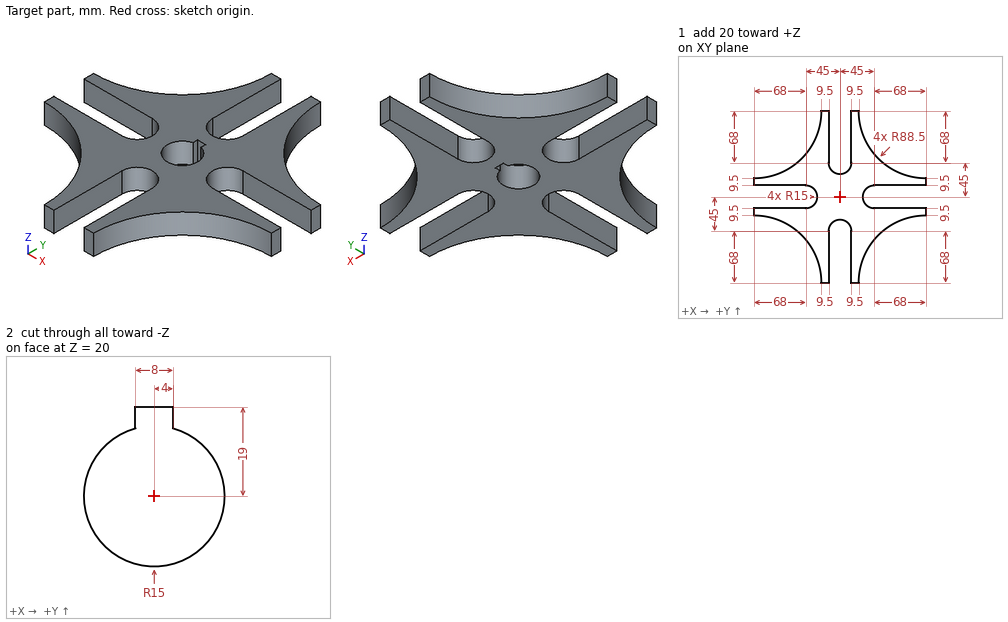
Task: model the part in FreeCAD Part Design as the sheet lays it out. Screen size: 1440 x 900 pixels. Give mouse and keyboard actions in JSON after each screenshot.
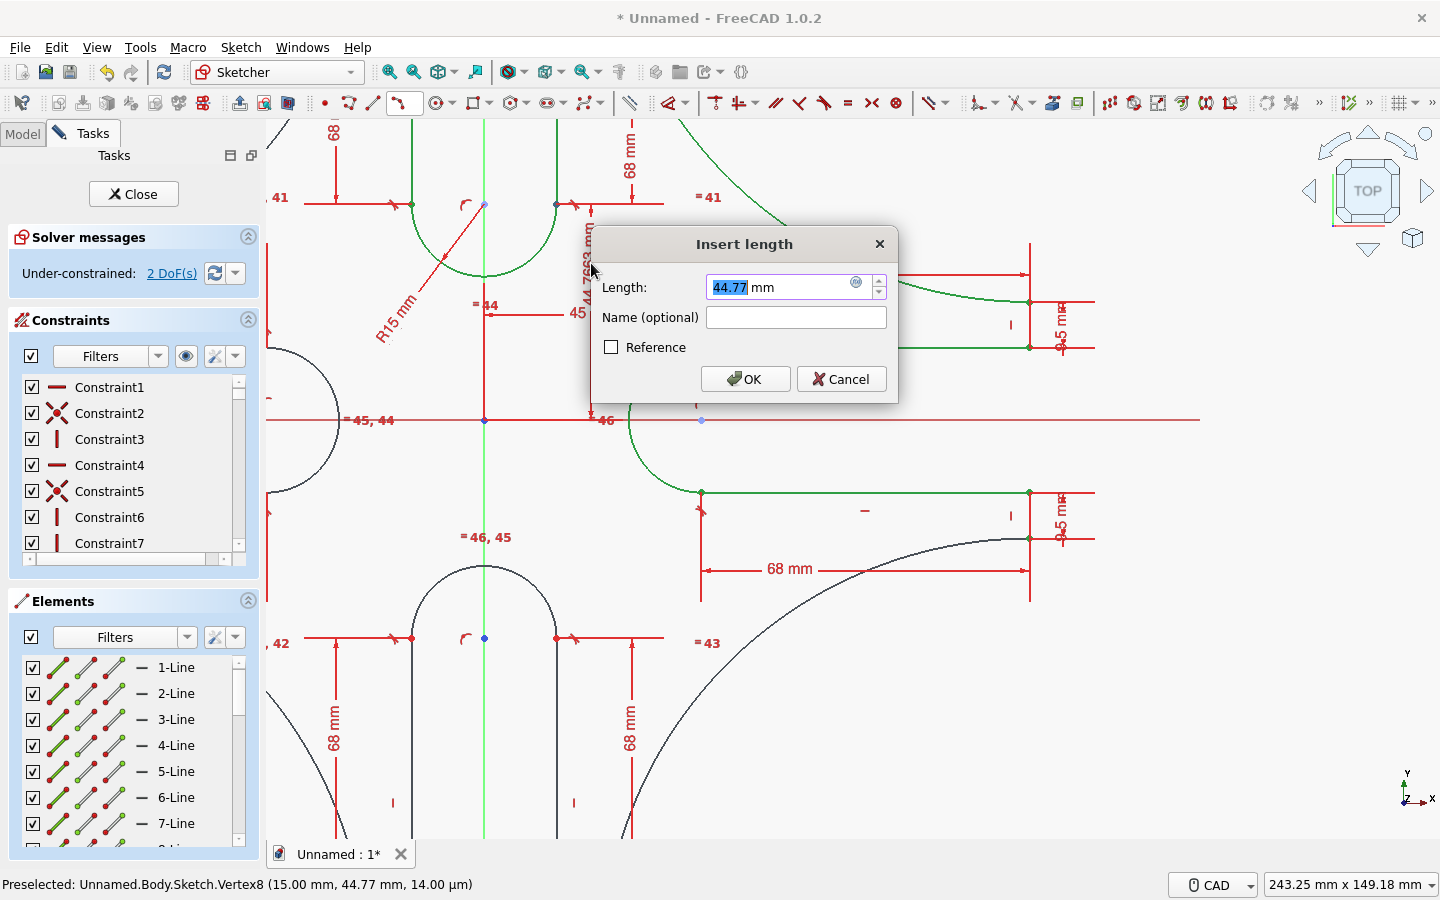
{"action": "type", "text": "45"}
{"action": "key", "text": "Return"}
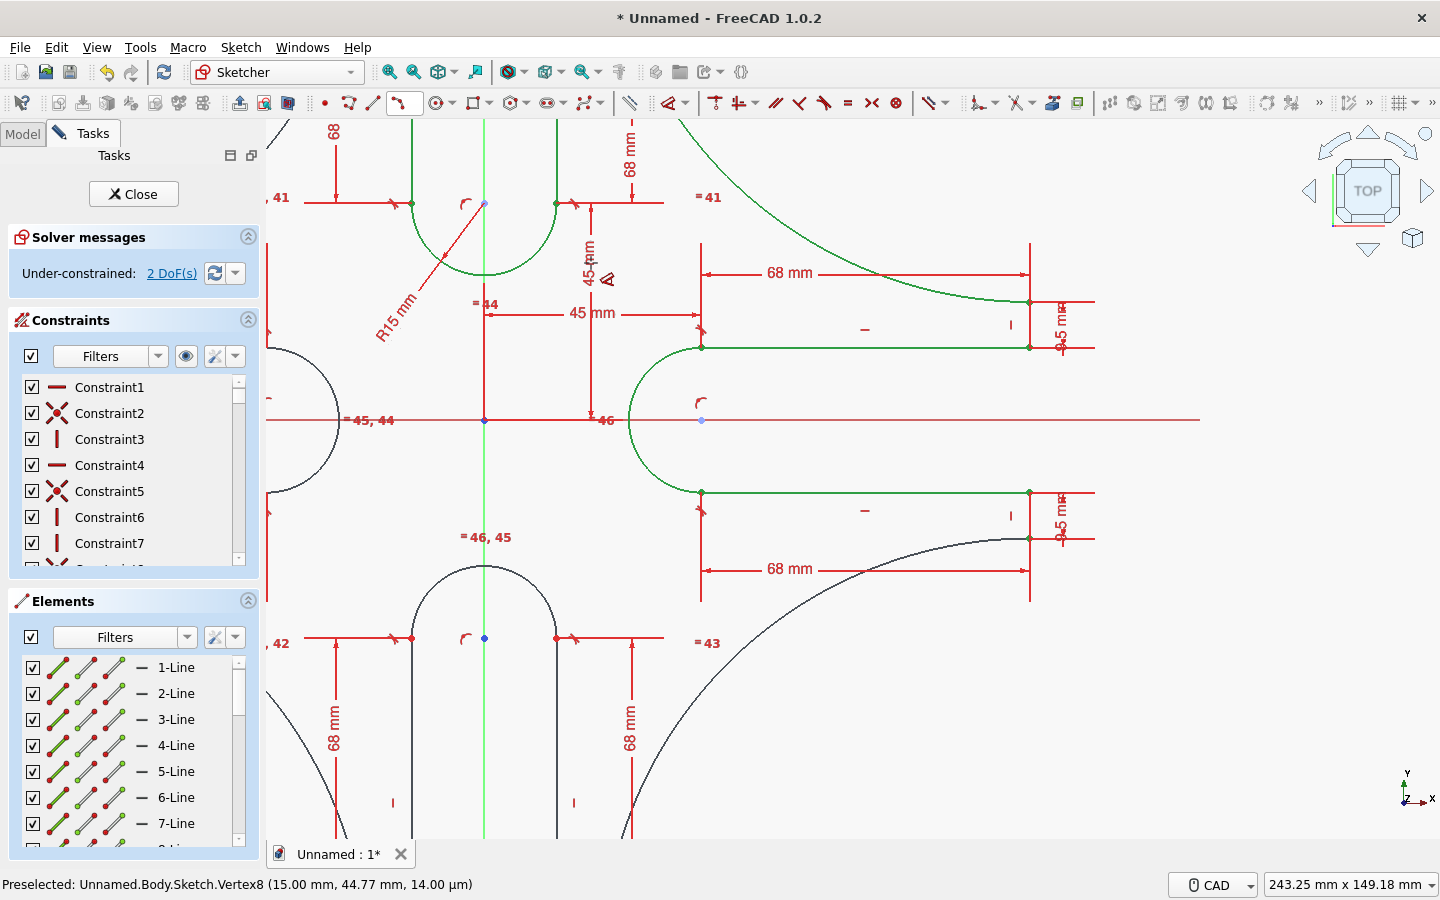
{"action": "scroll", "coordinate": [1030, 527], "scroll_direction": "down", "scroll_amount": 4}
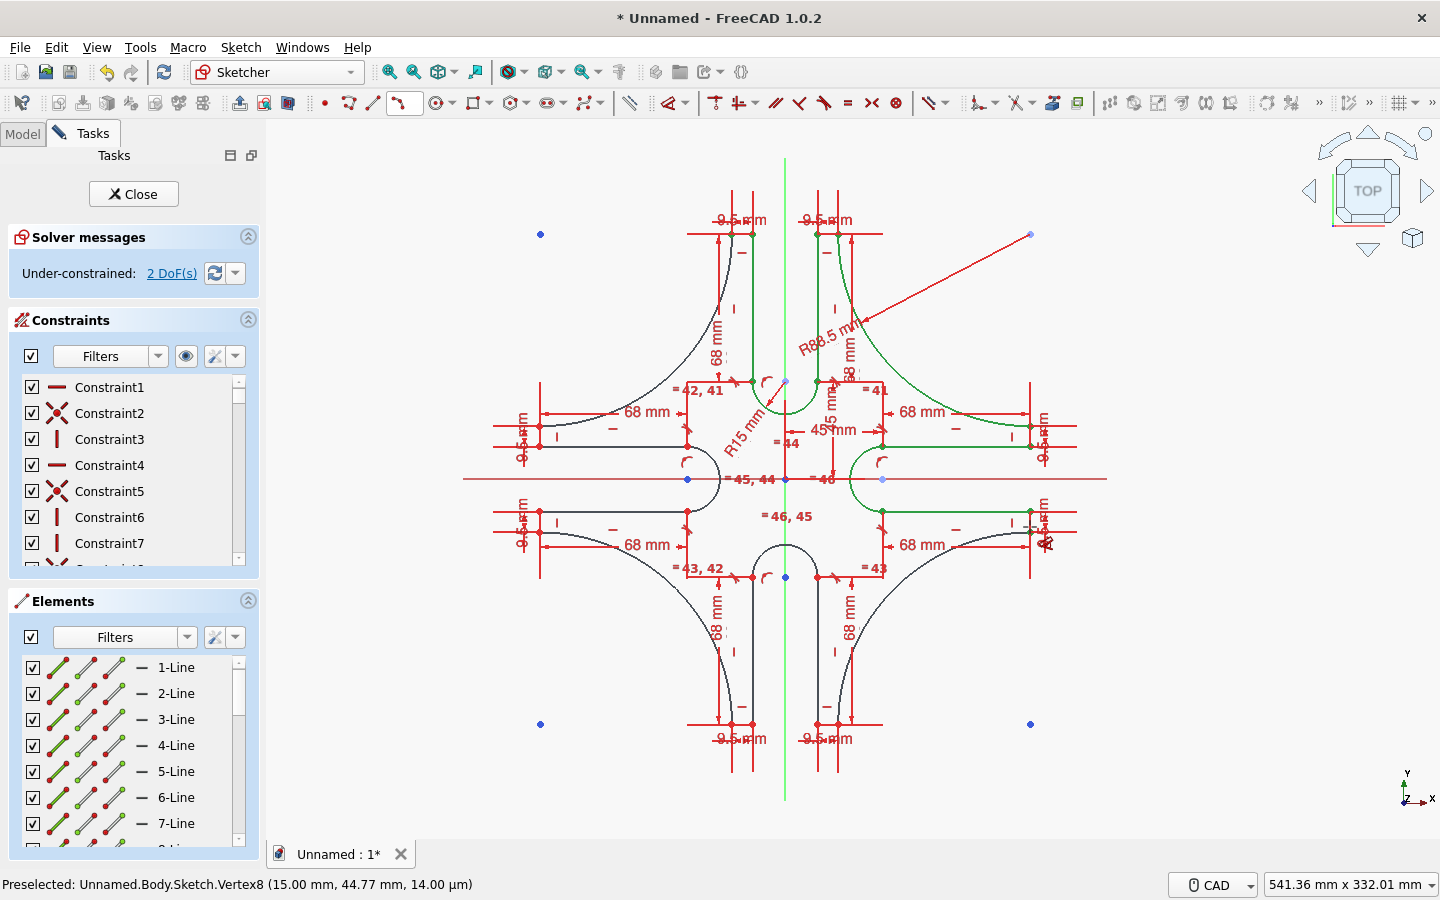
{"action": "left_click", "coordinate": [687, 447]}
{"action": "left_click", "coordinate": [736, 413]}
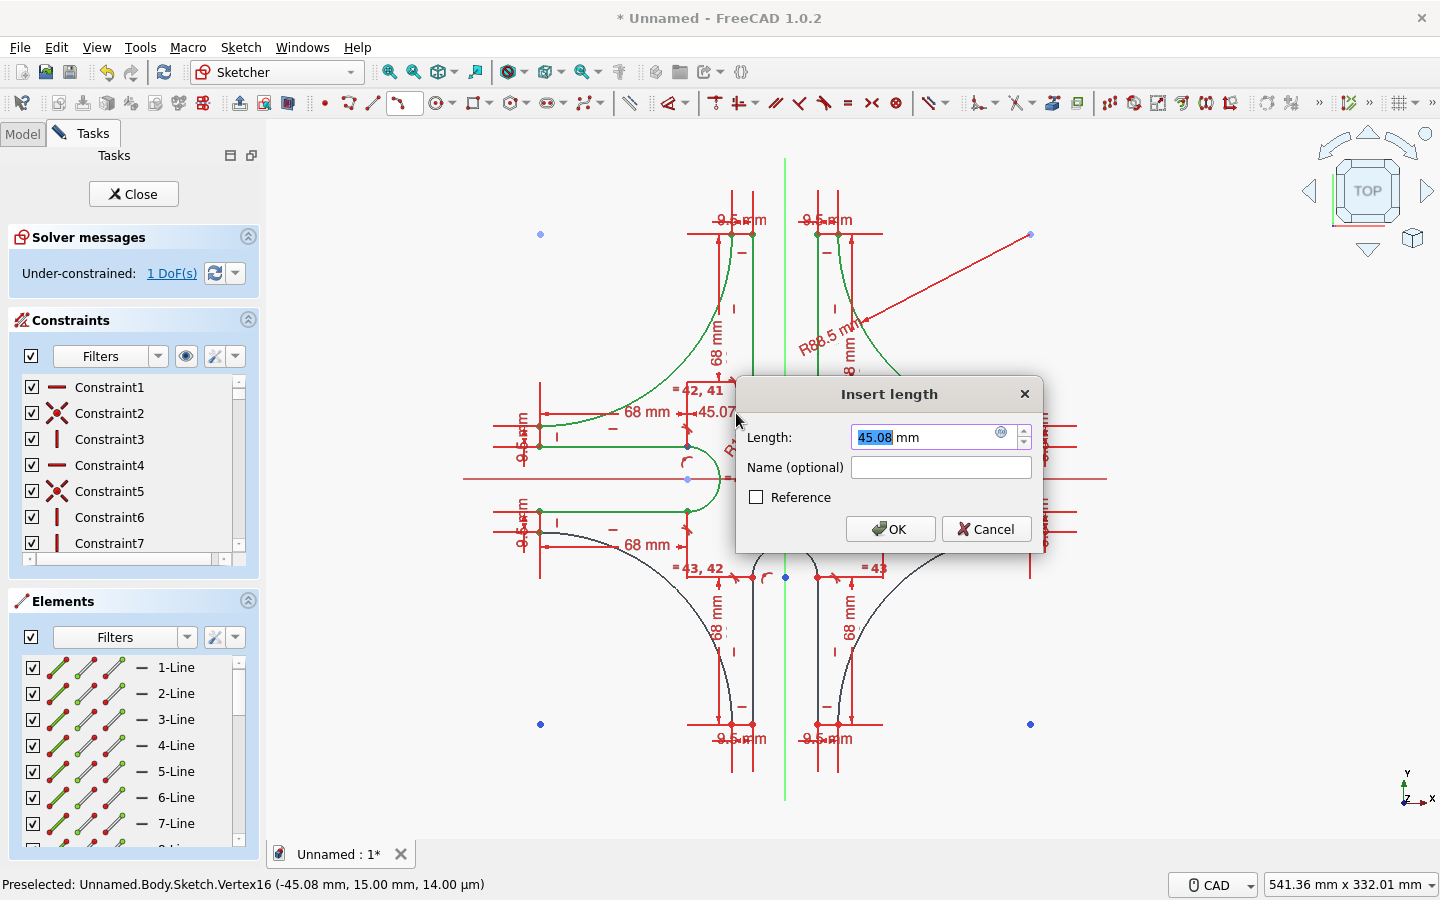
{"action": "type", "text": "45"}
{"action": "key", "text": "Return"}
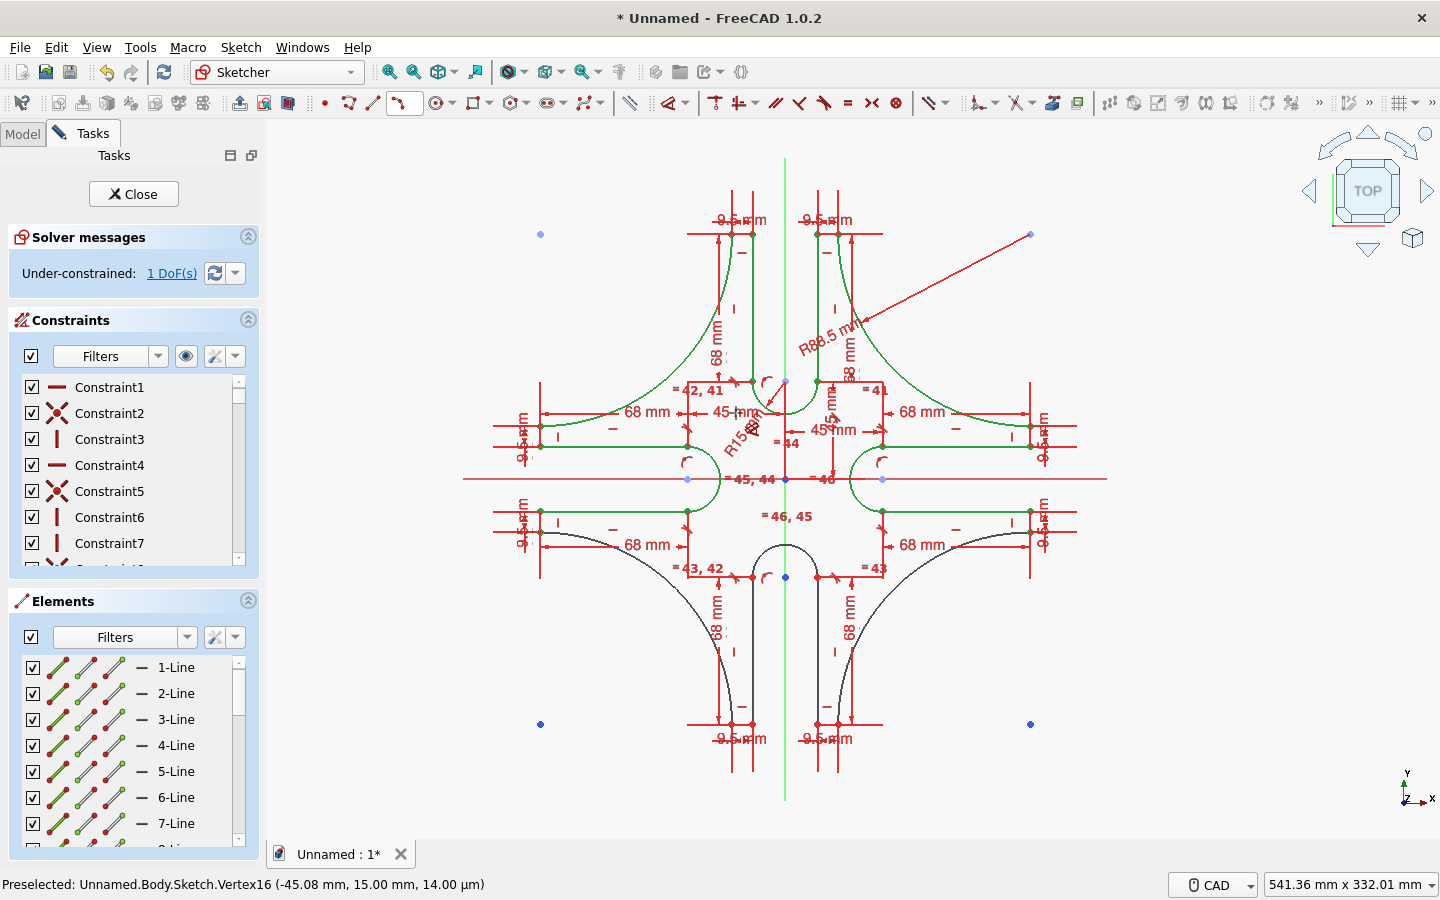
{"action": "left_click", "coordinate": [753, 577]}
{"action": "left_click", "coordinate": [719, 528]}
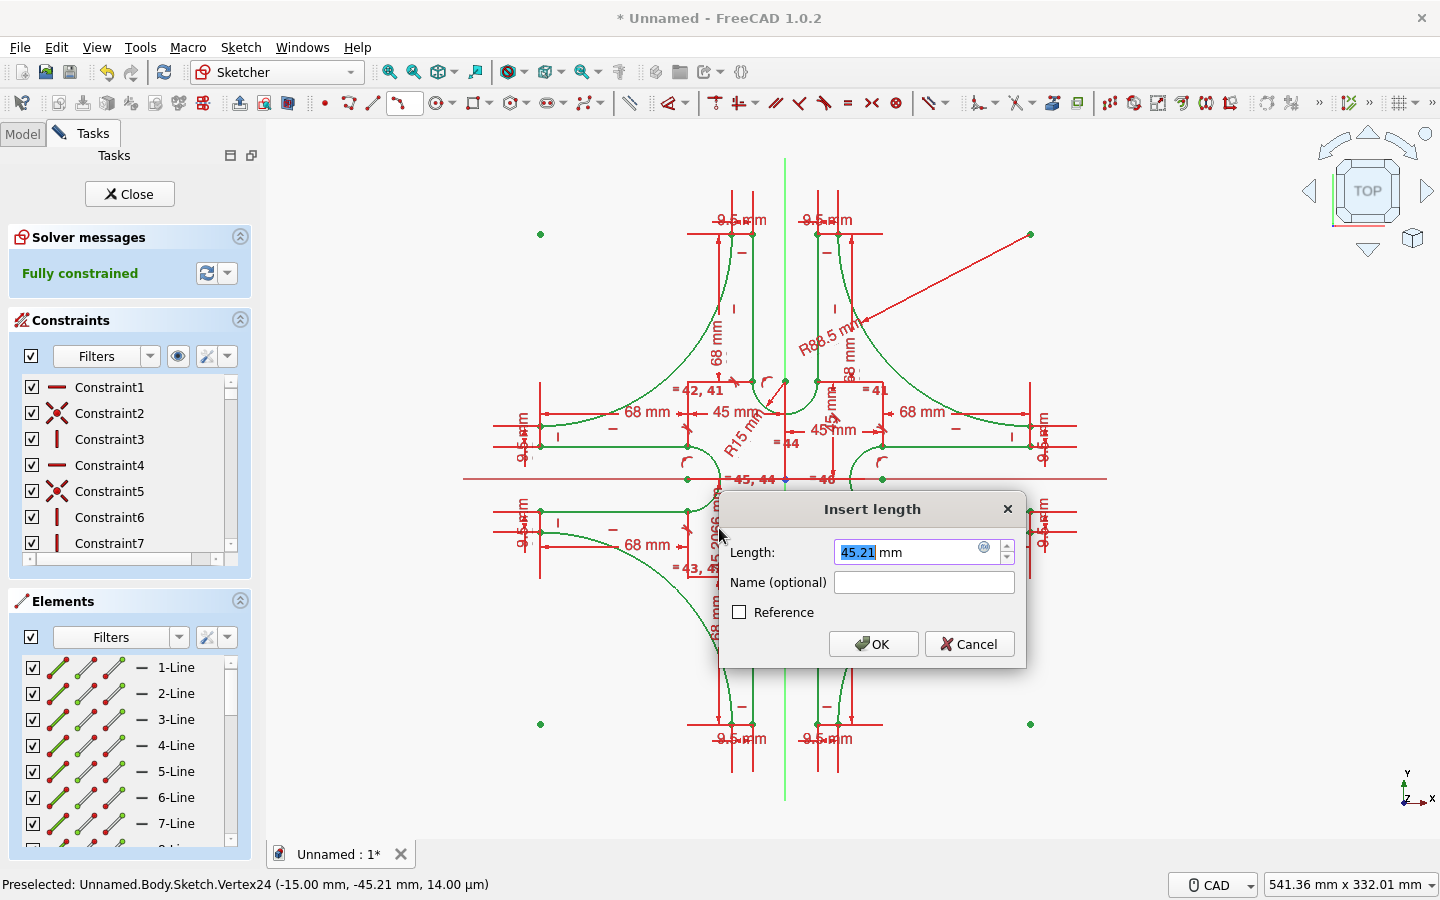
{"action": "type", "text": "45"}
{"action": "key", "text": "Return"}
{"action": "key", "text": "Escape"}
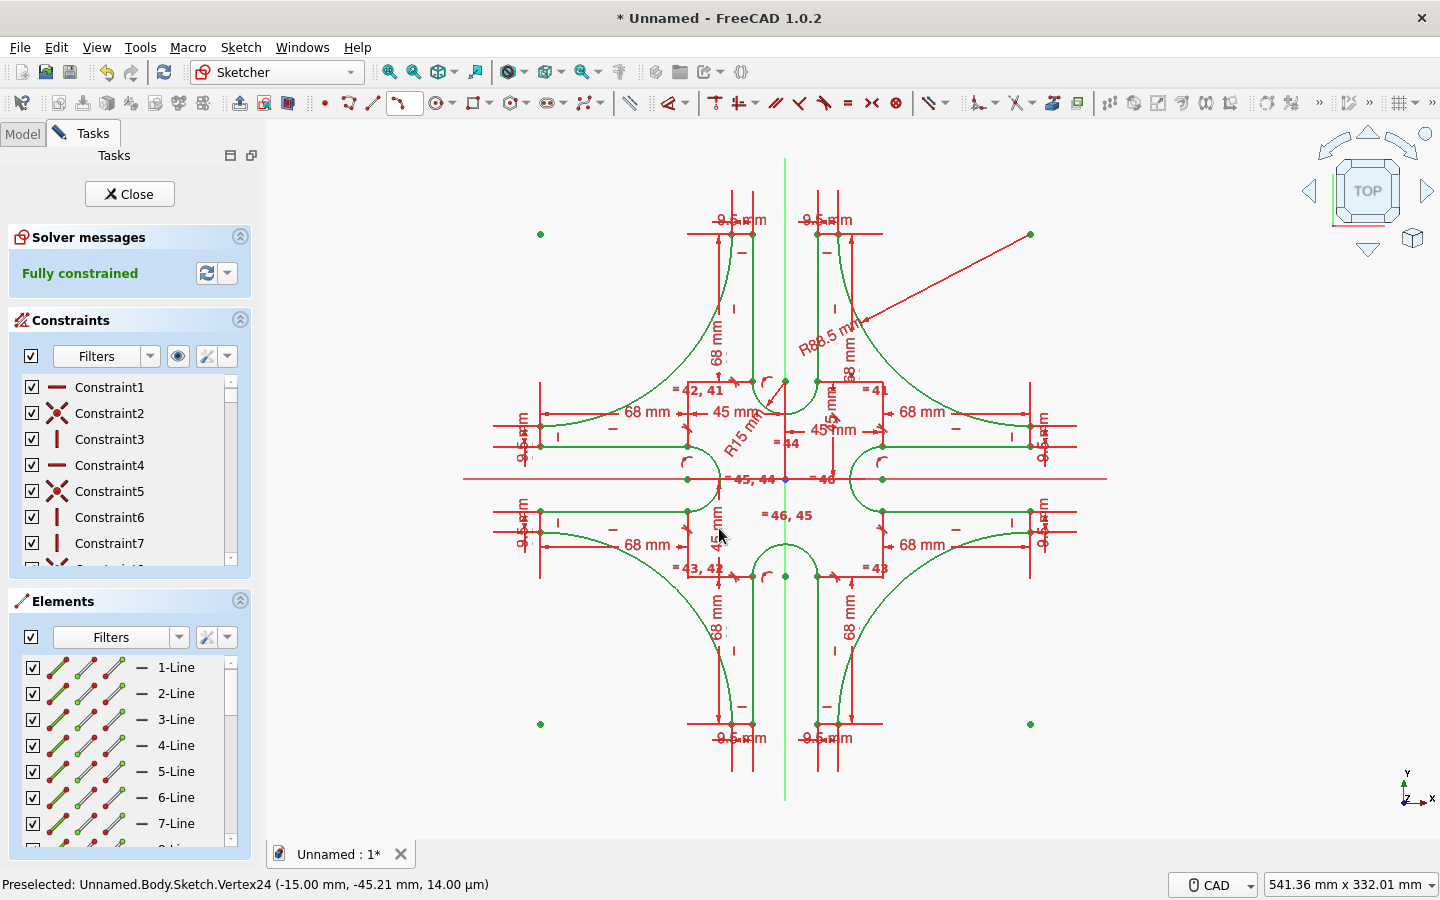
{"action": "left_click", "coordinate": [130, 194]}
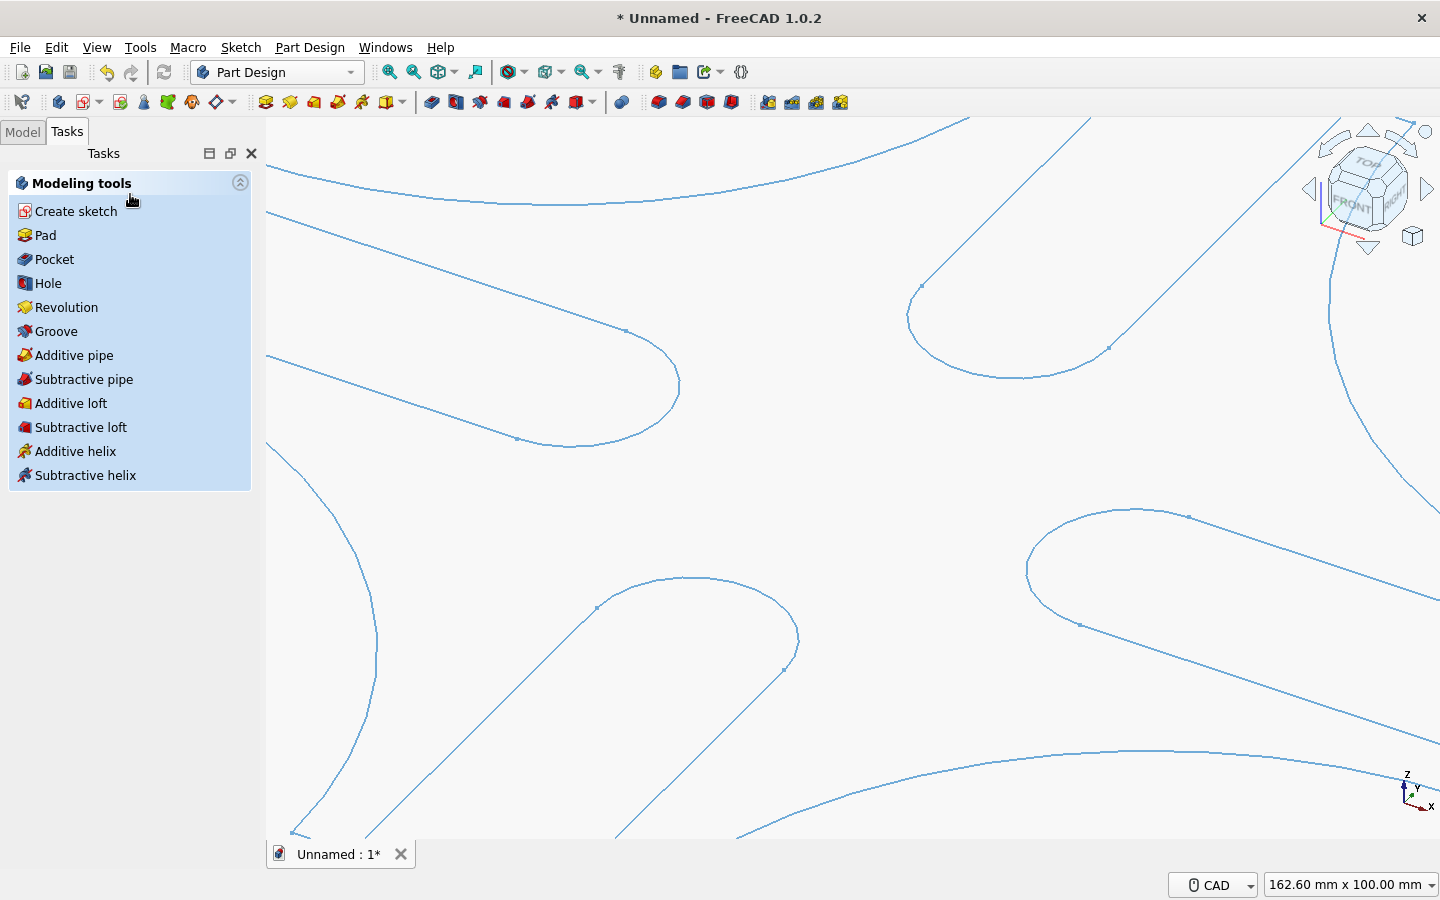
{"action": "left_click", "coordinate": [266, 102]}